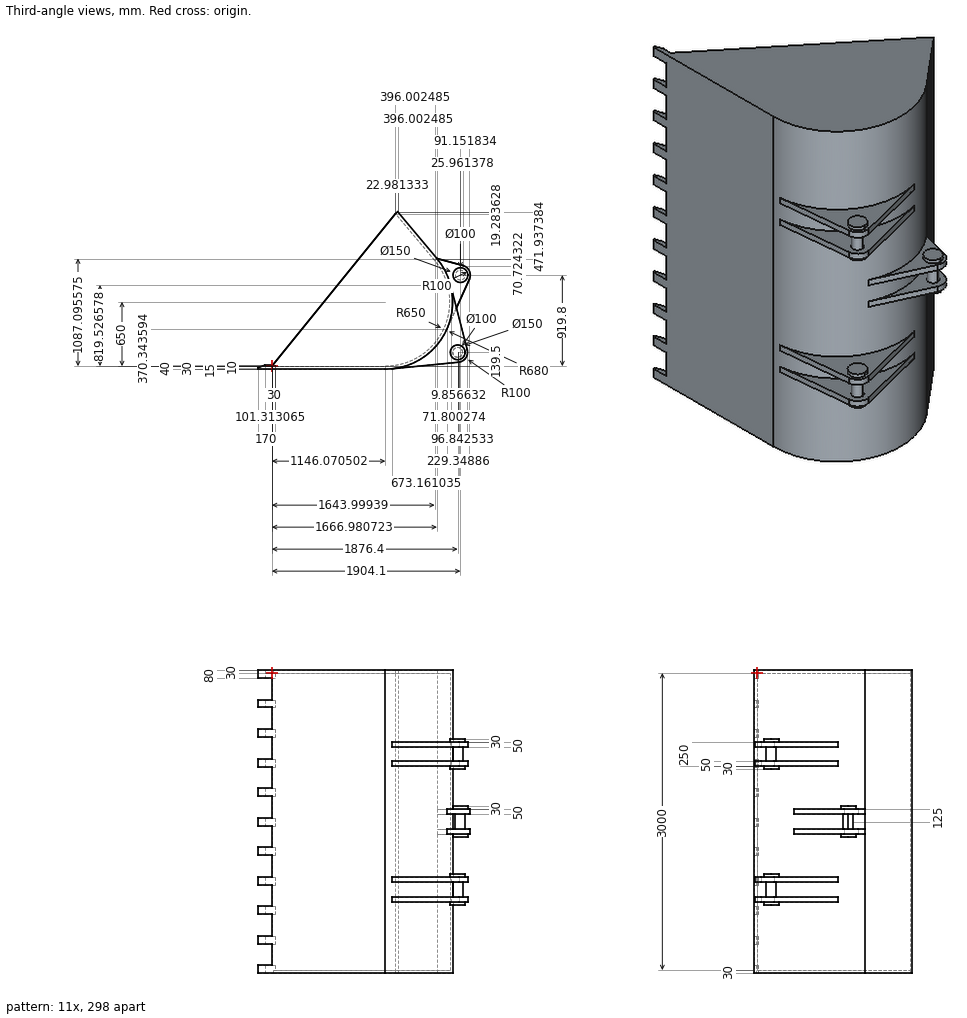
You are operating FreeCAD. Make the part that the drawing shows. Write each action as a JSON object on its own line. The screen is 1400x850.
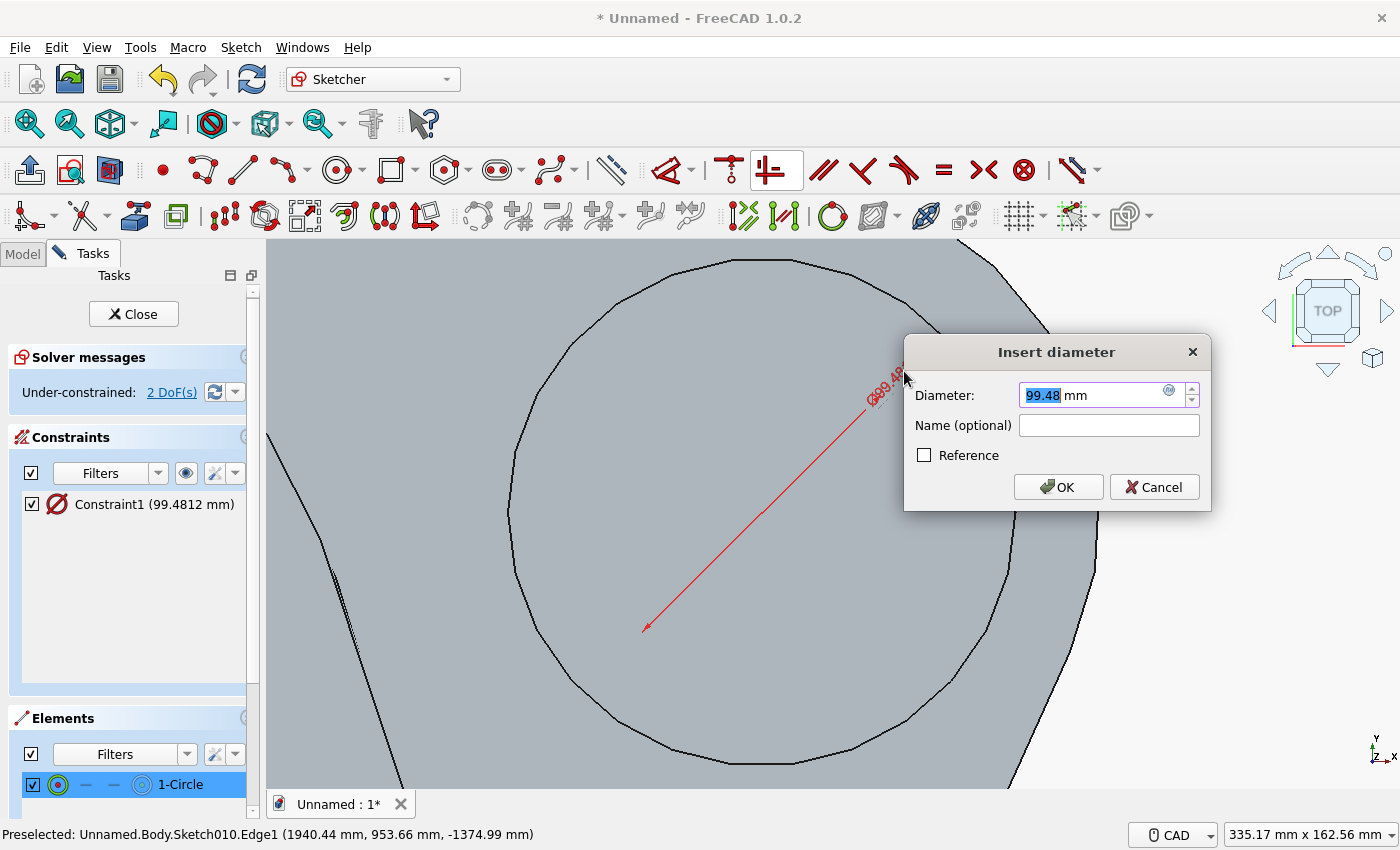
{"action": "type", "text": "100"}
{"action": "key", "text": "Return"}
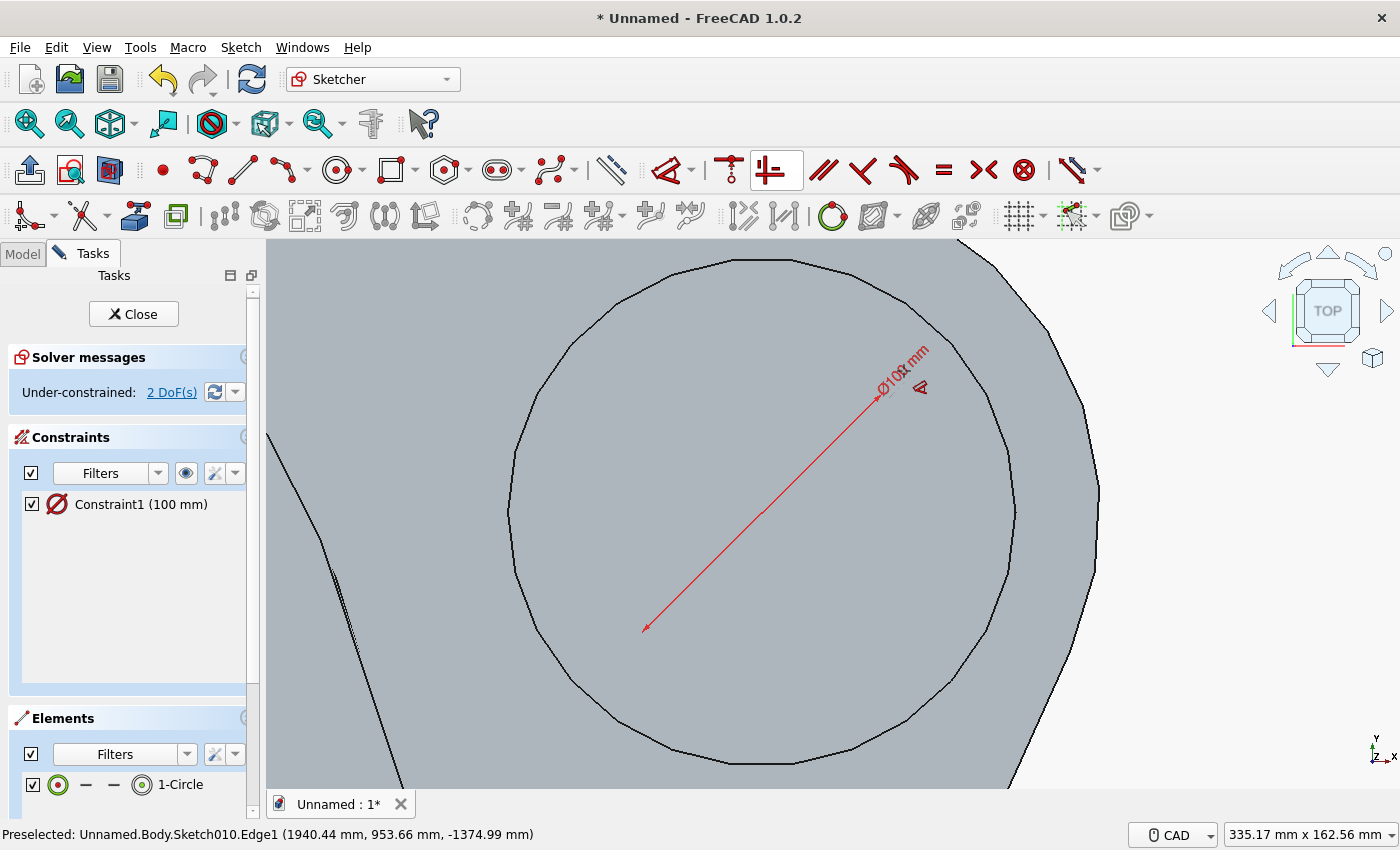
{"action": "left_click", "coordinate": [762, 513]}
{"action": "left_click", "coordinate": [796, 637]}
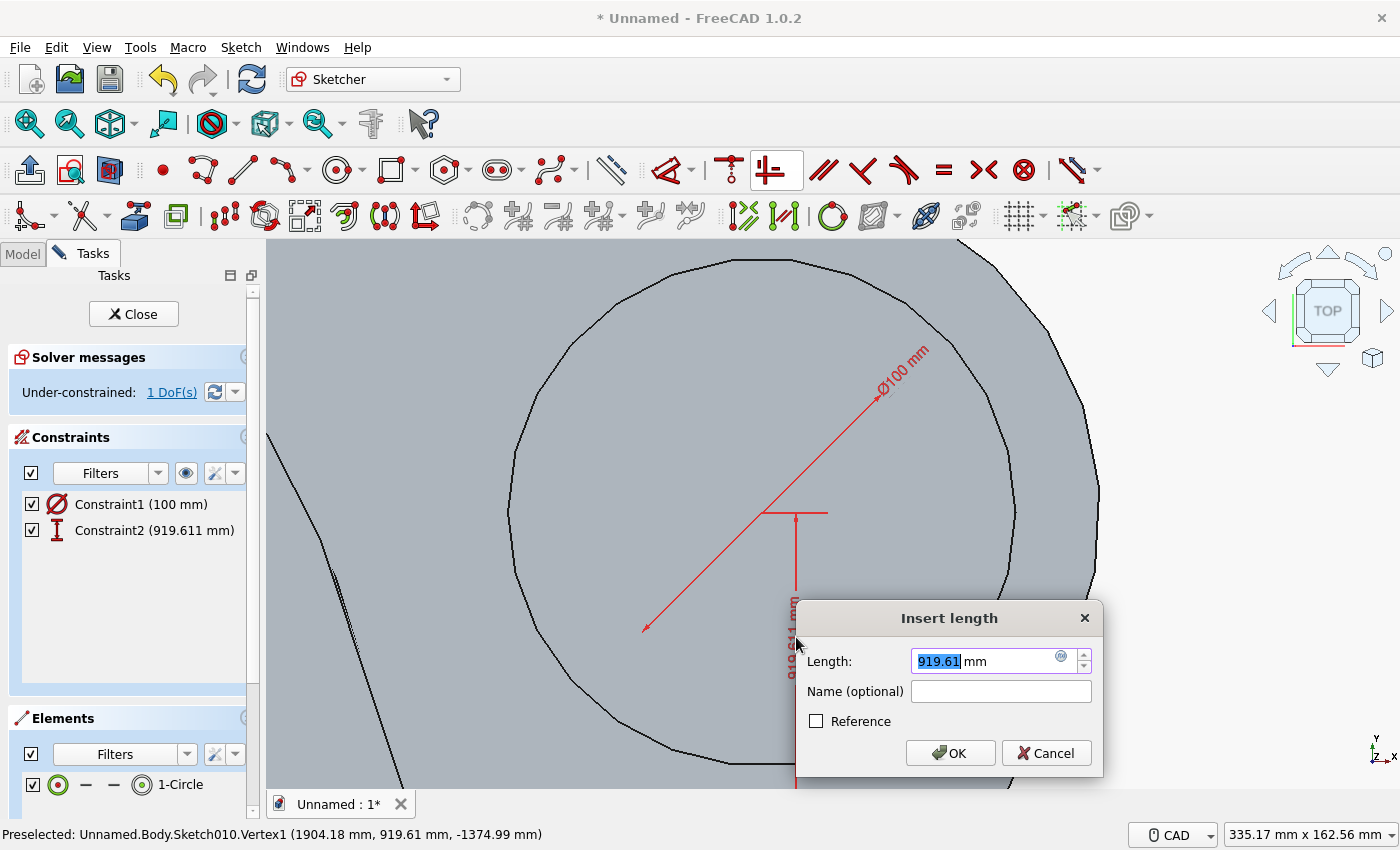
{"action": "type", "text": "919.8"}
{"action": "key", "text": "Return"}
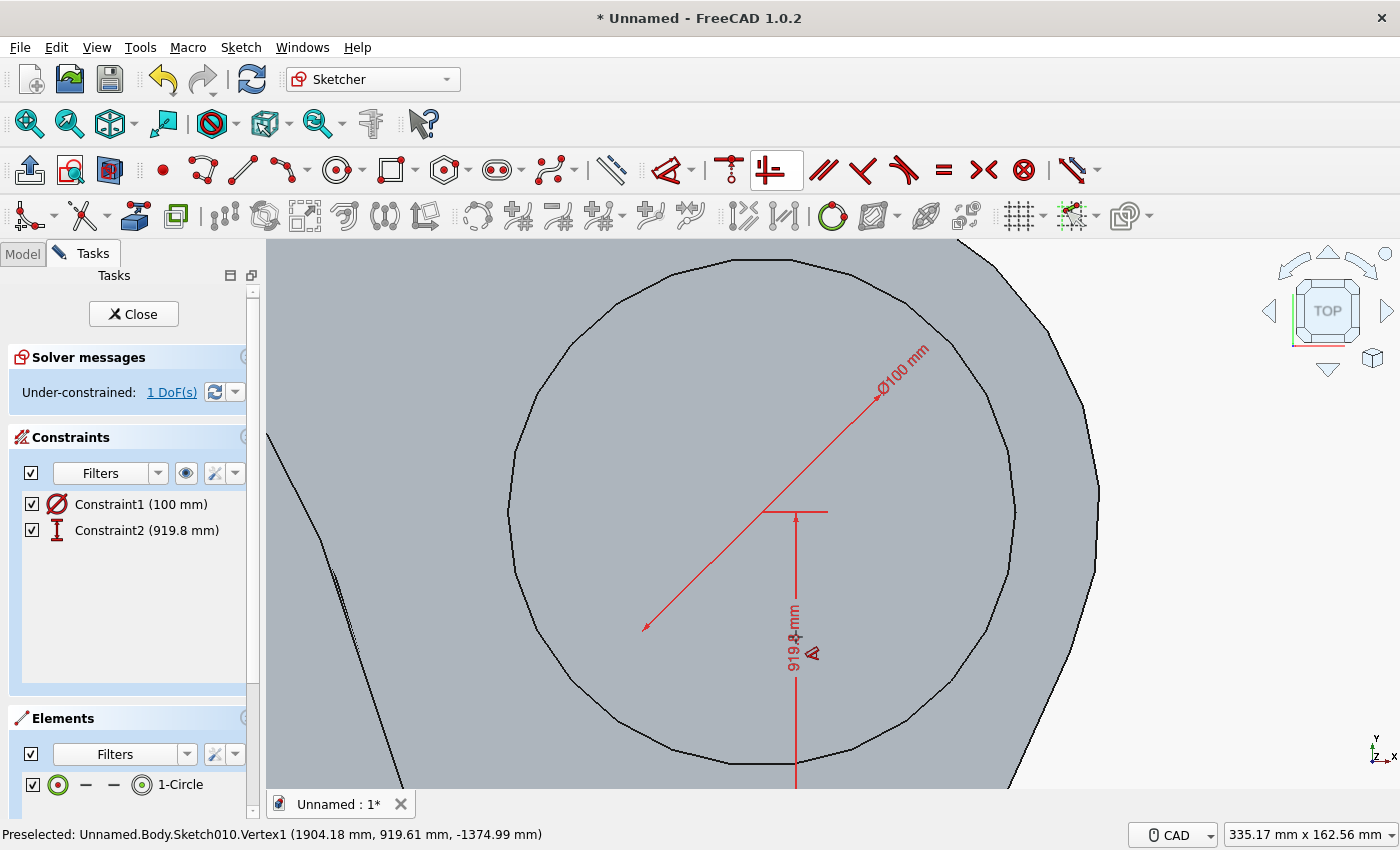
{"action": "left_click", "coordinate": [762, 512]}
{"action": "left_click", "coordinate": [528, 478]}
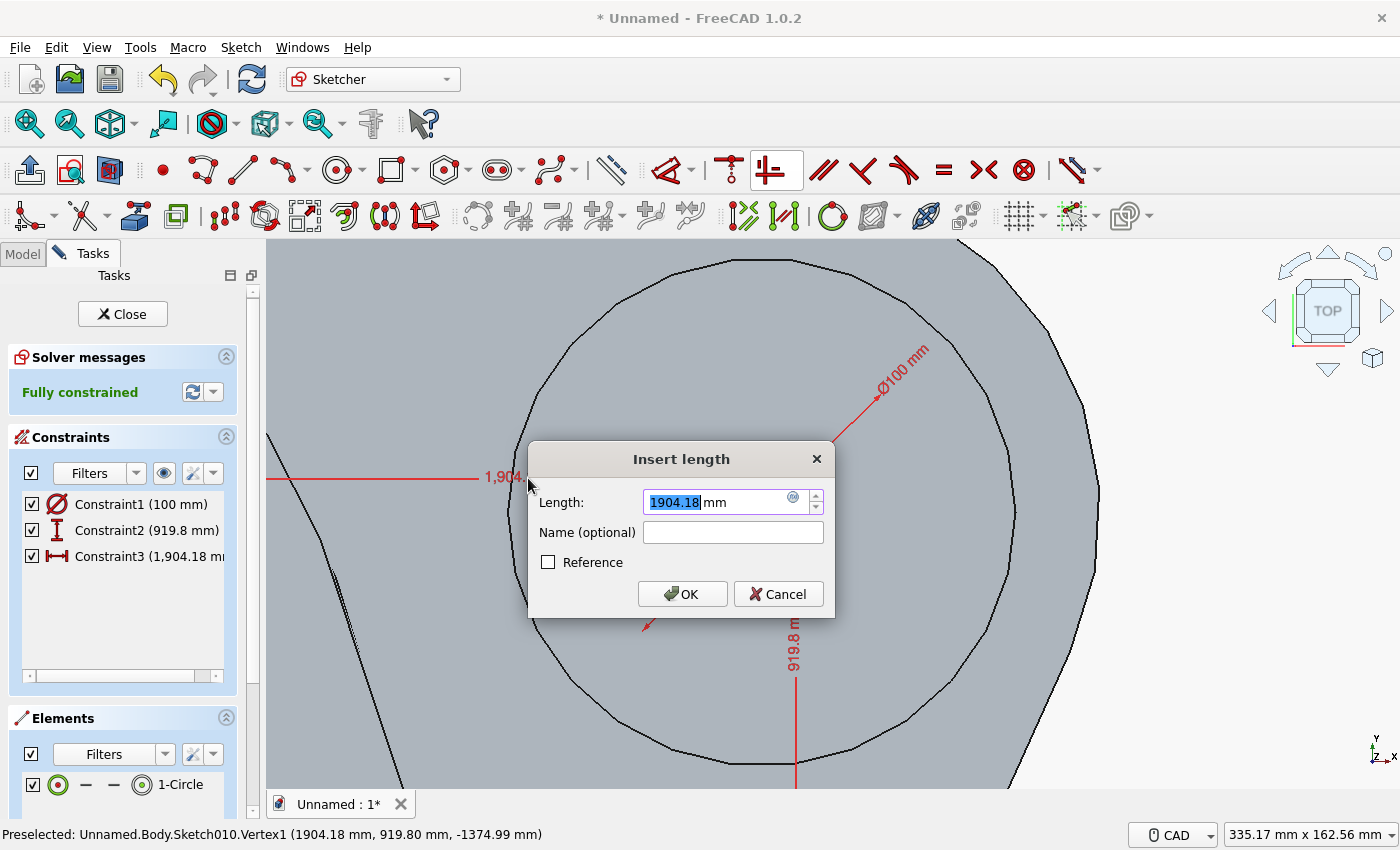
{"action": "type", "text": "1904.1"}
{"action": "key", "text": "Return"}
{"action": "key", "text": "Escape"}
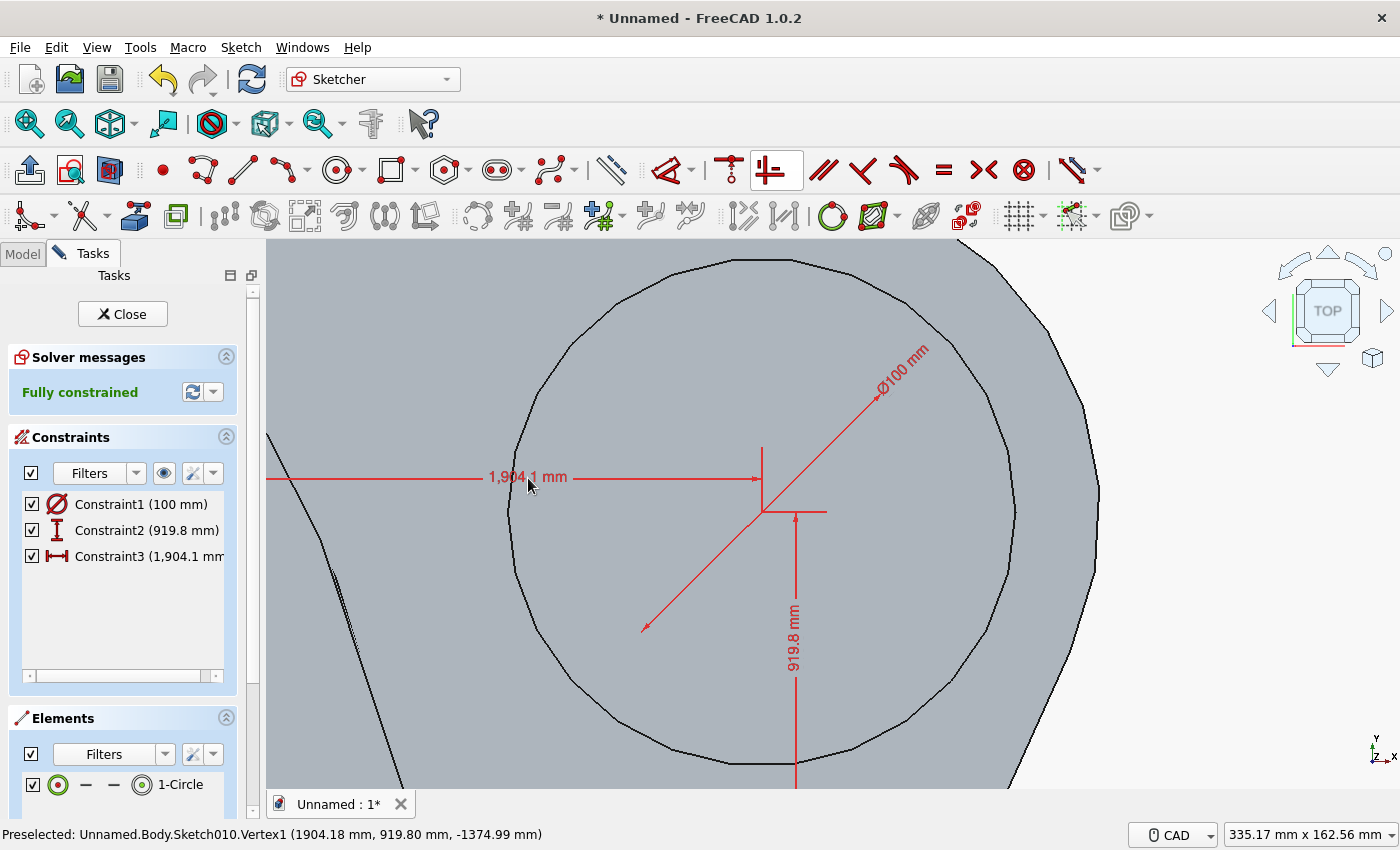
{"action": "left_click", "coordinate": [123, 314]}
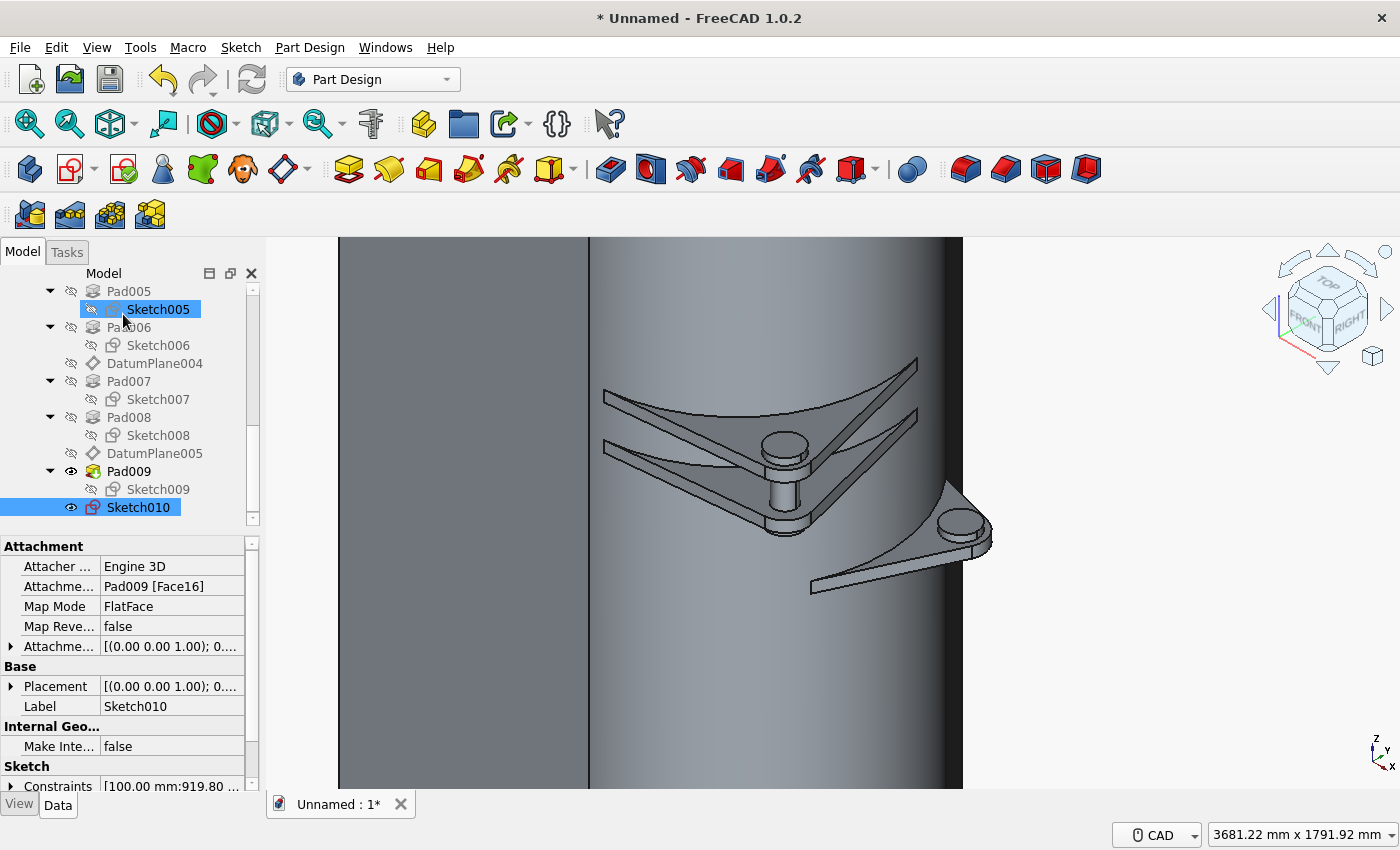
{"action": "left_click", "coordinate": [350, 170]}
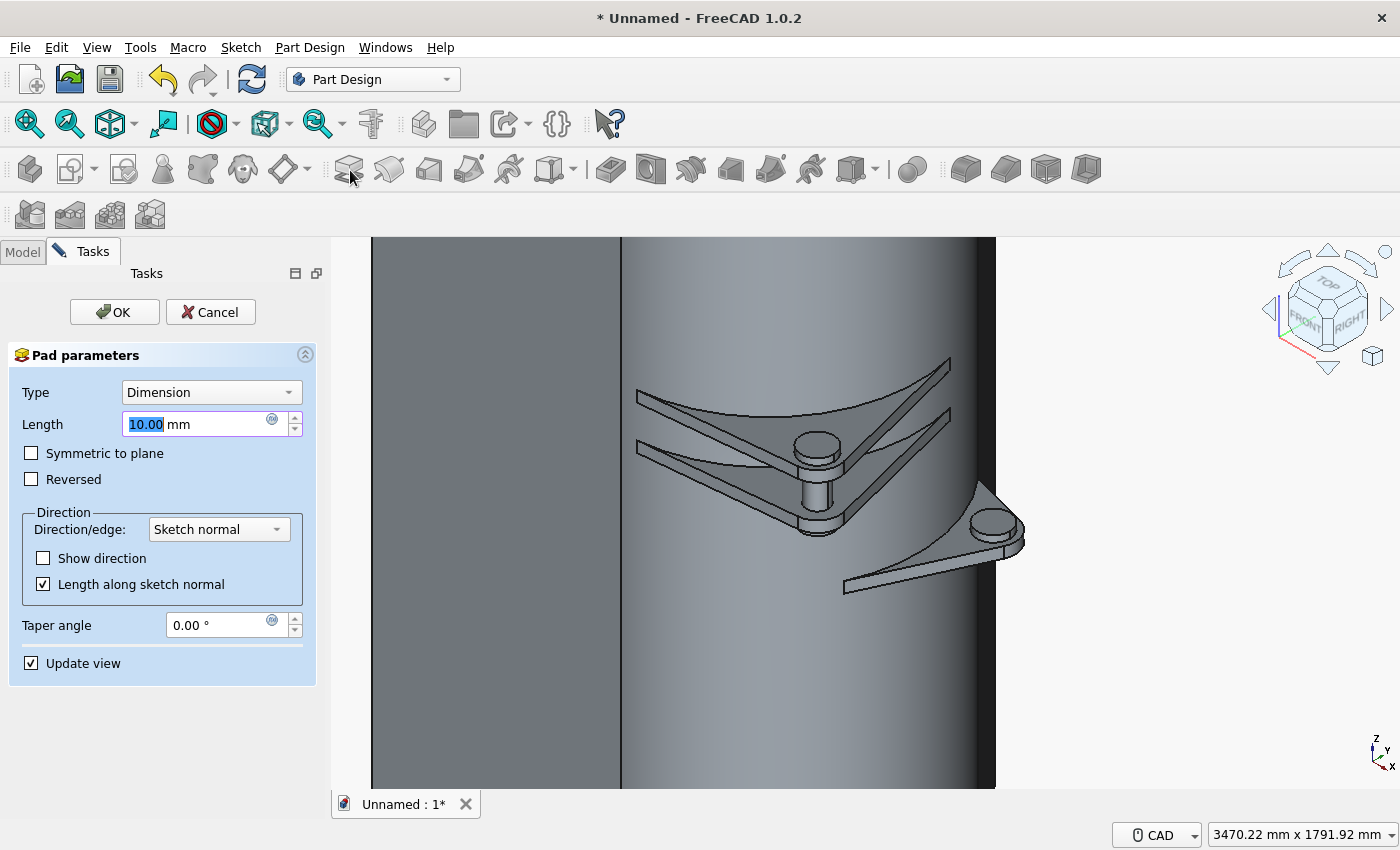
{"action": "type", "text": "125"}
{"action": "key", "text": "Tab"}